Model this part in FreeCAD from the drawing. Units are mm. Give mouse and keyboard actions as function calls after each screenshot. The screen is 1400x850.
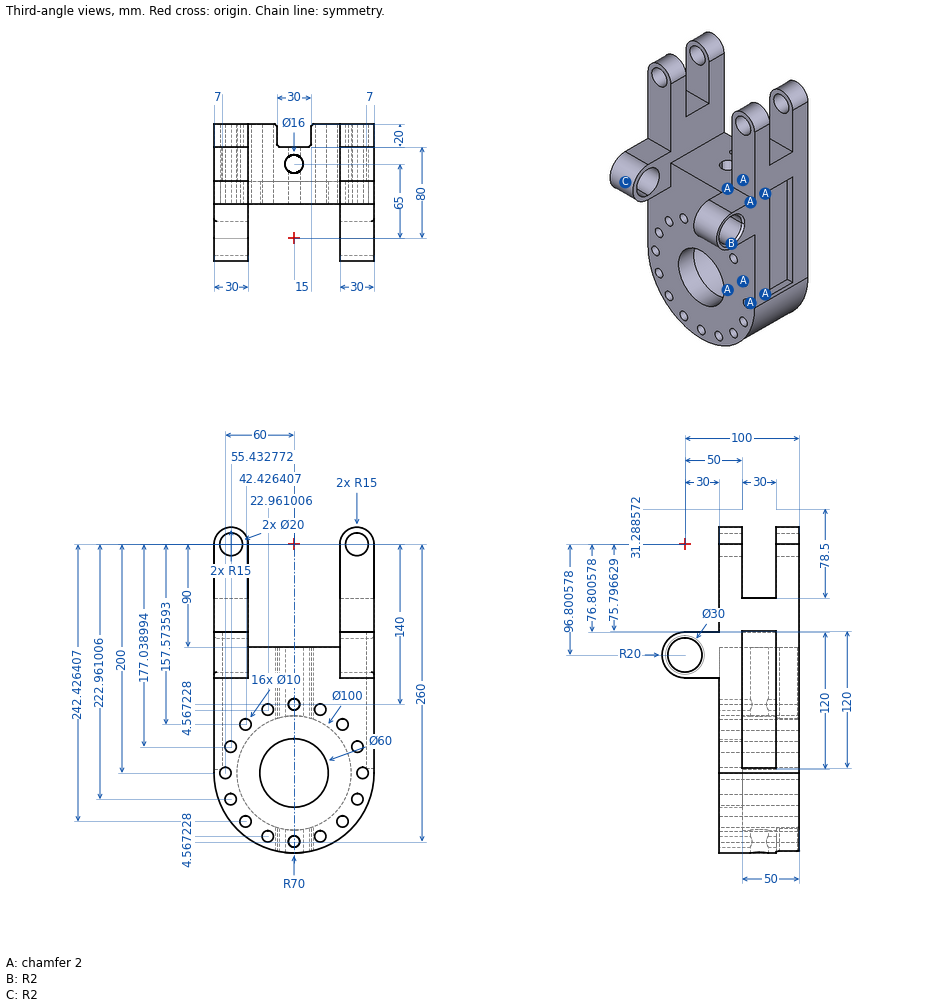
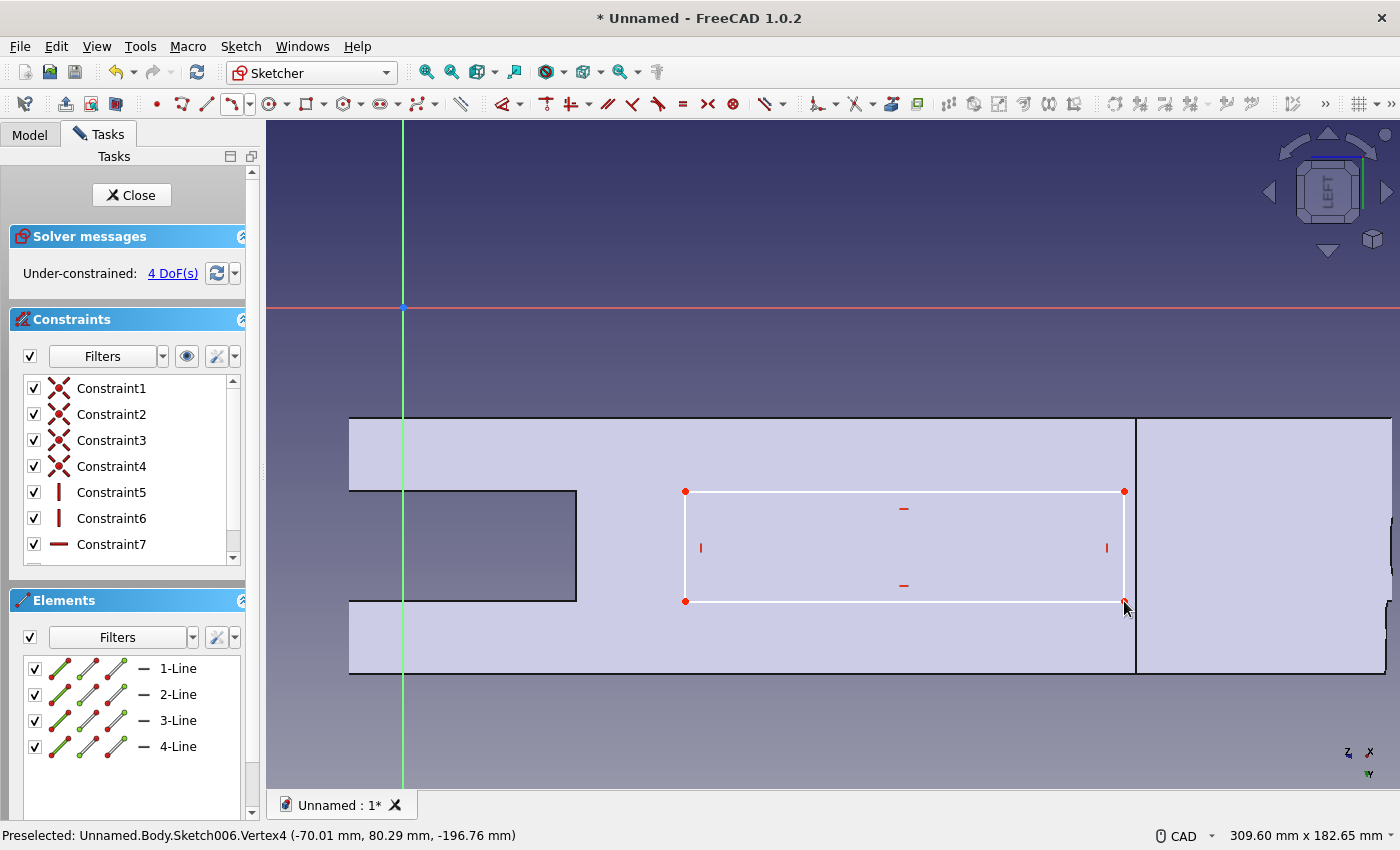
key(d)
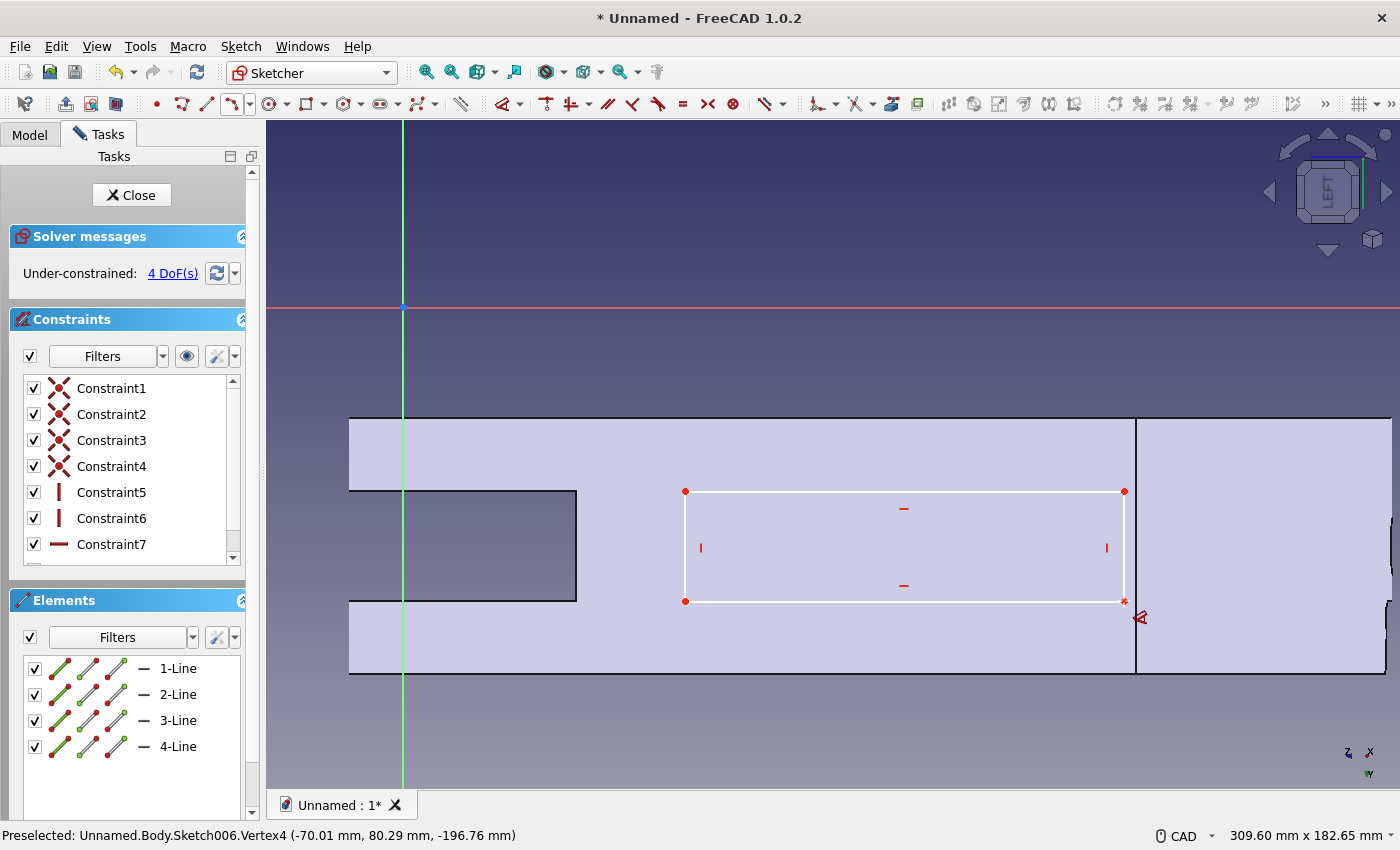
click(685, 525)
click(651, 547)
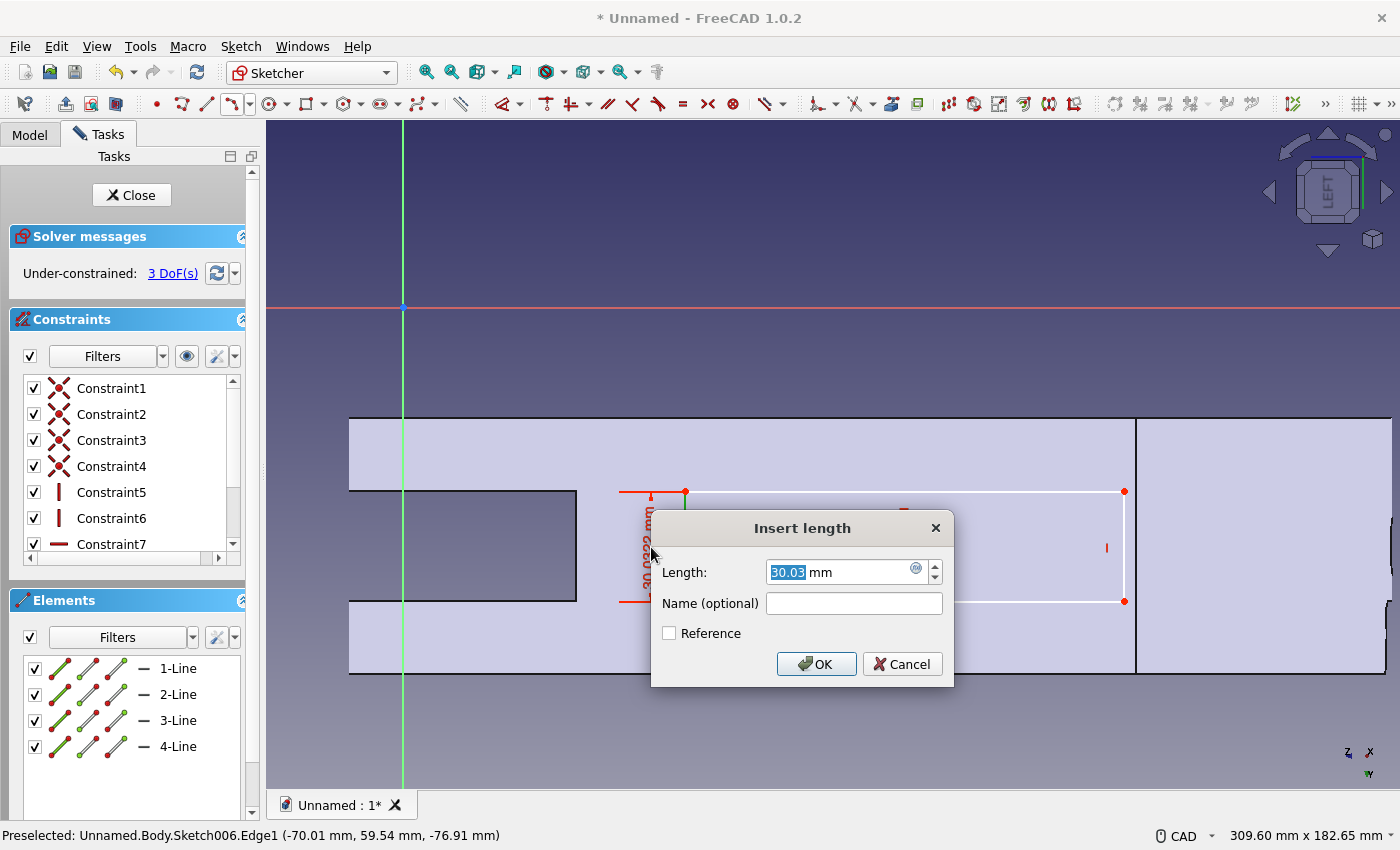
text(30)
key(Return)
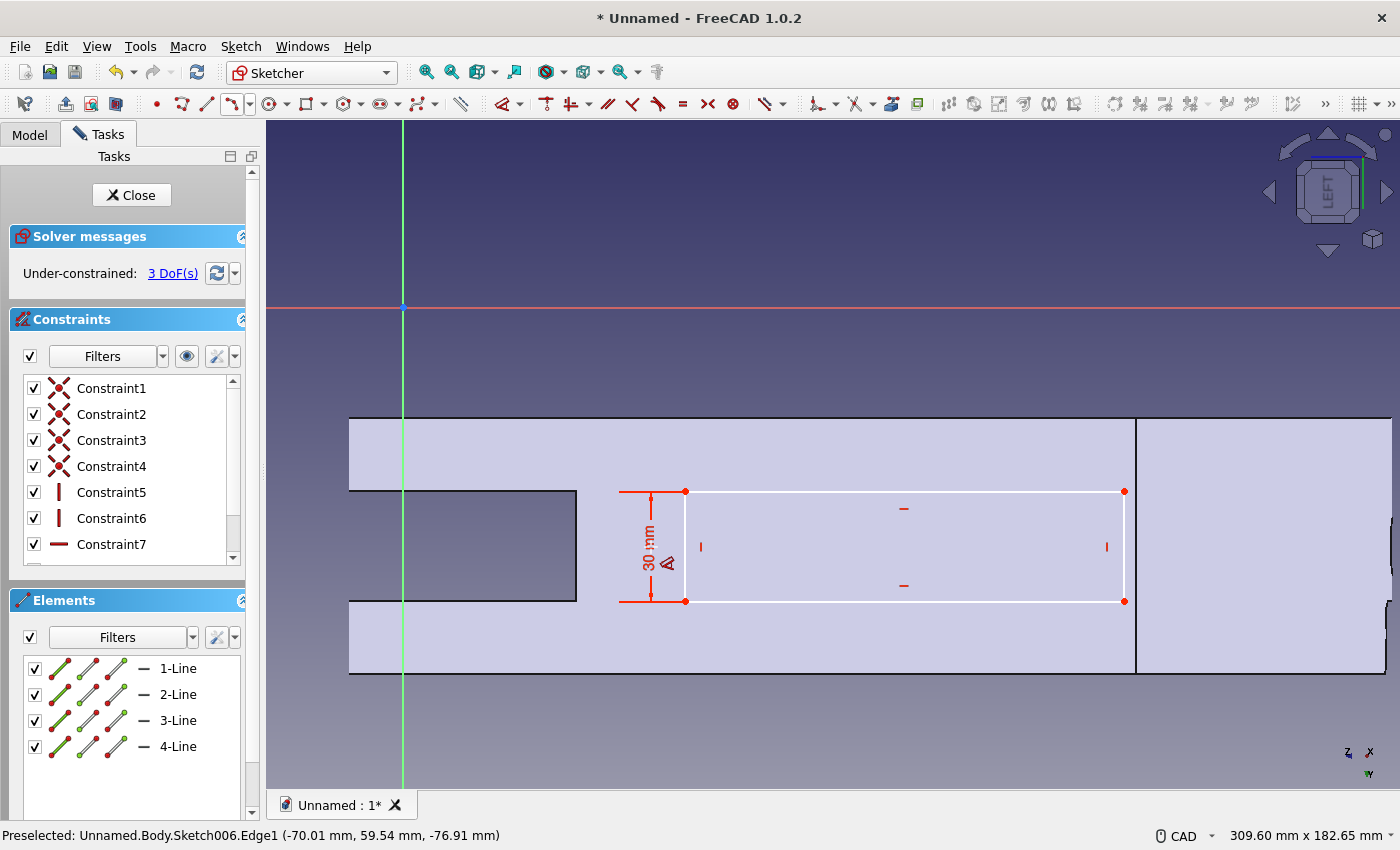
click(817, 602)
click(904, 636)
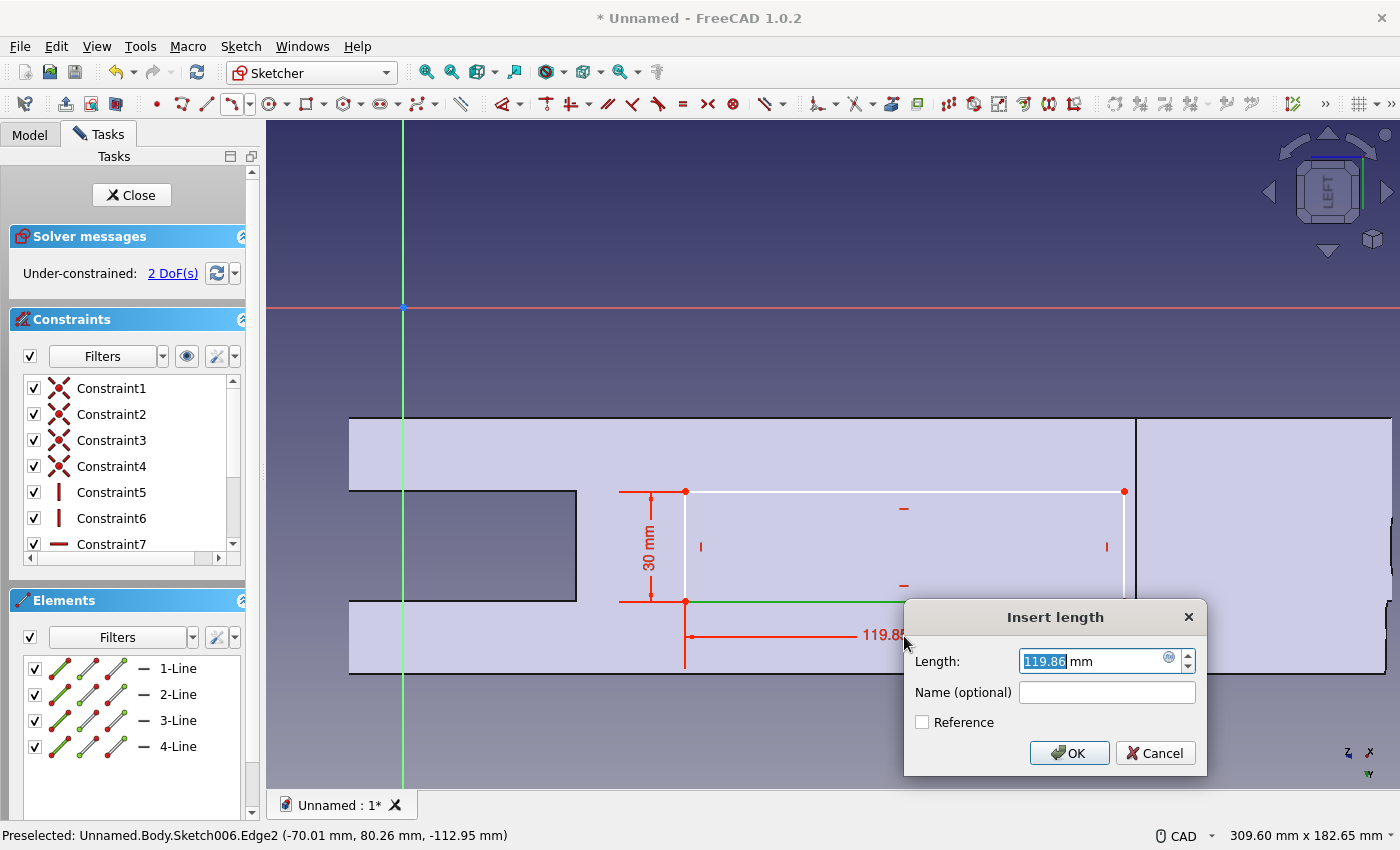
text(120)
key(Return)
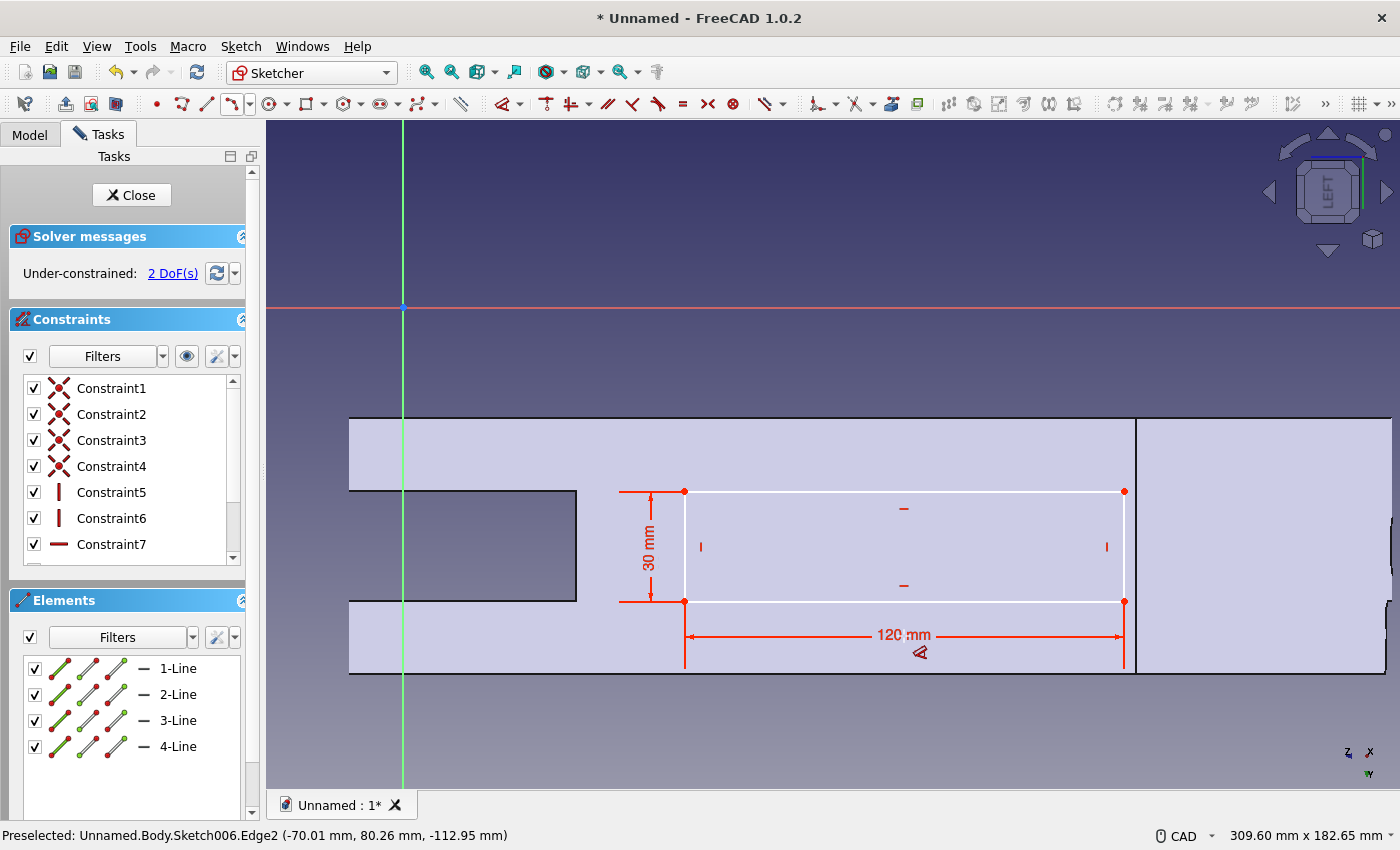
click(685, 492)
click(369, 400)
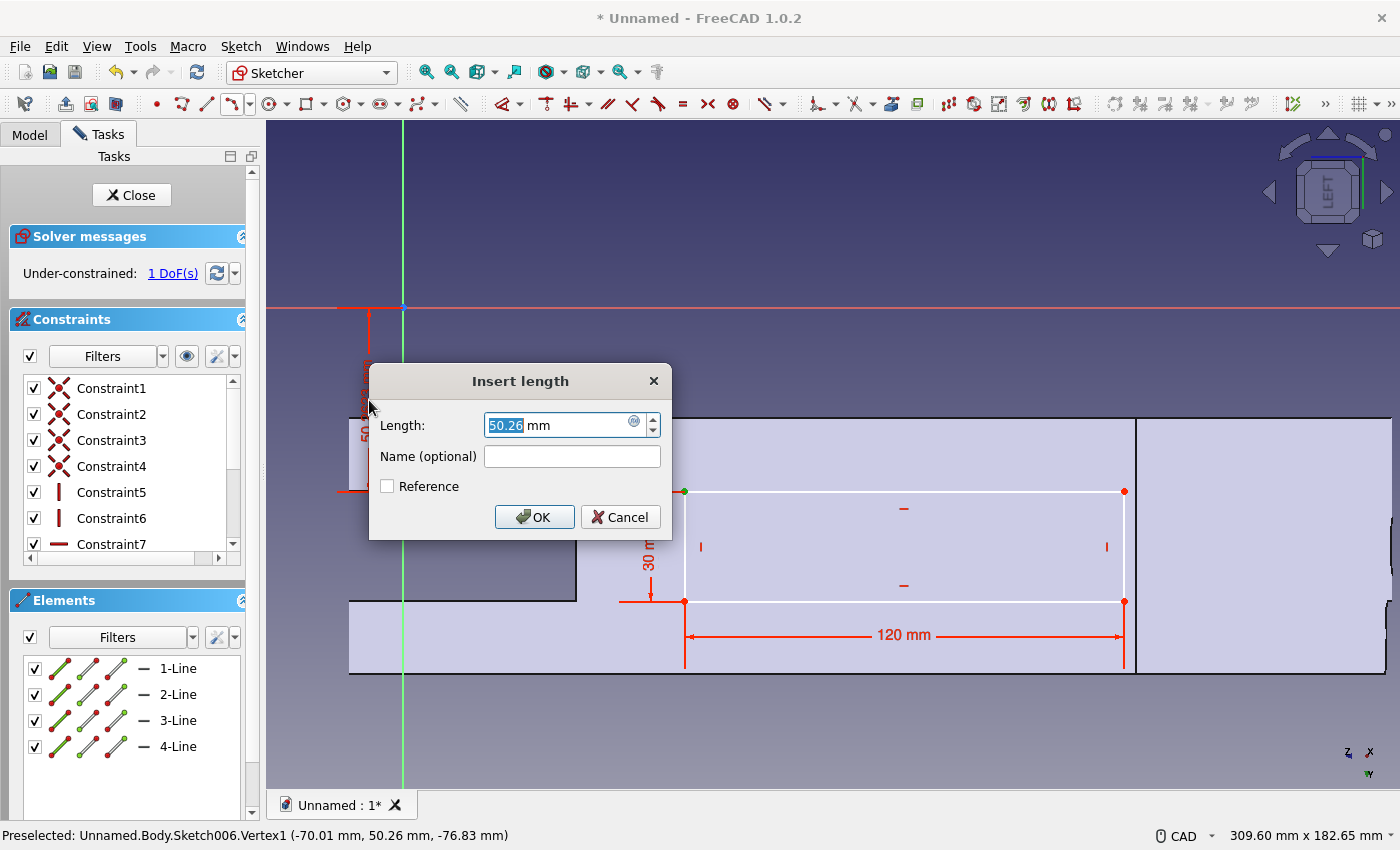
text(50)
key(Return)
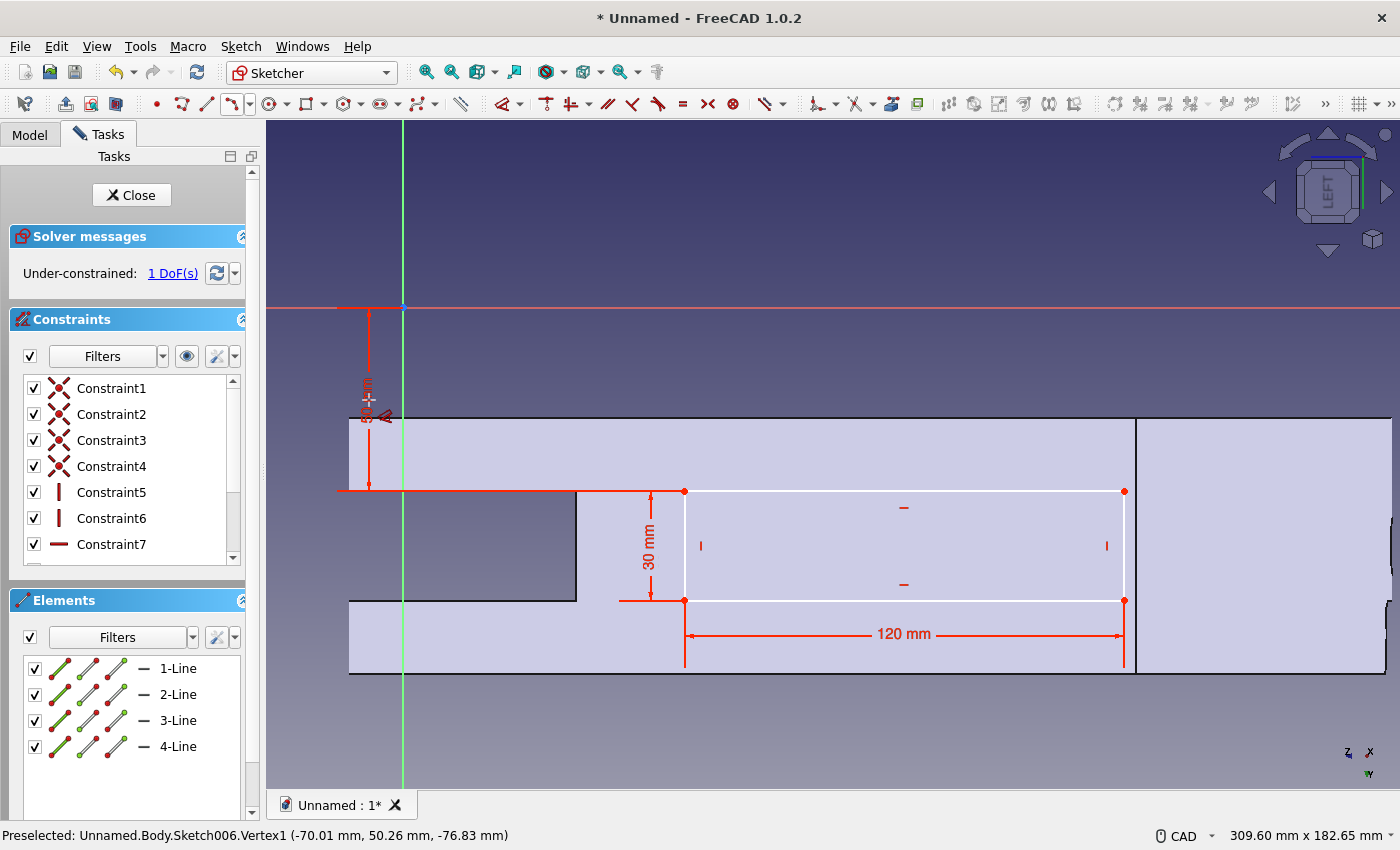
click(685, 491)
click(544, 274)